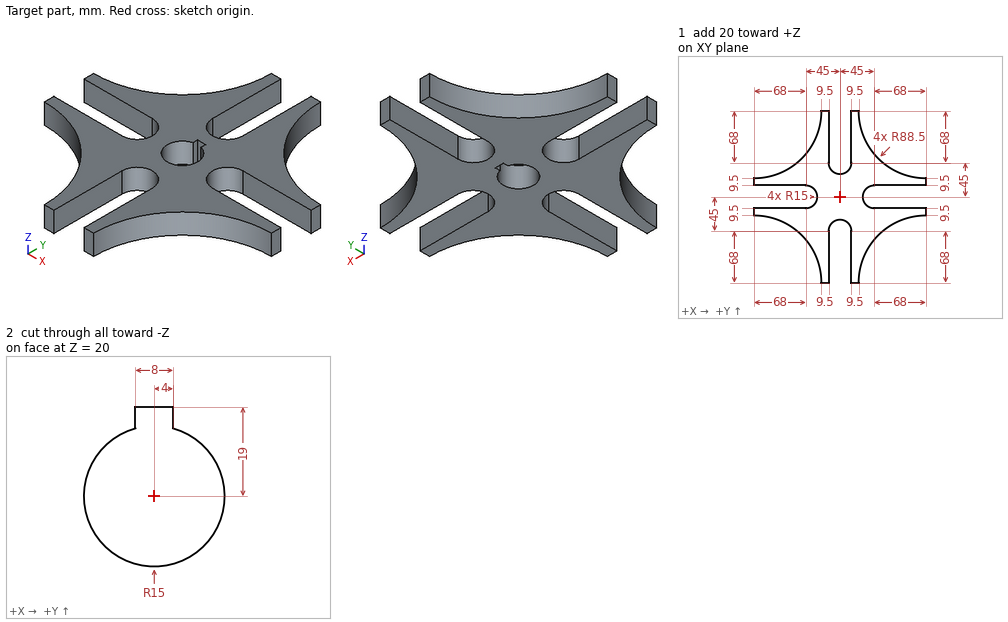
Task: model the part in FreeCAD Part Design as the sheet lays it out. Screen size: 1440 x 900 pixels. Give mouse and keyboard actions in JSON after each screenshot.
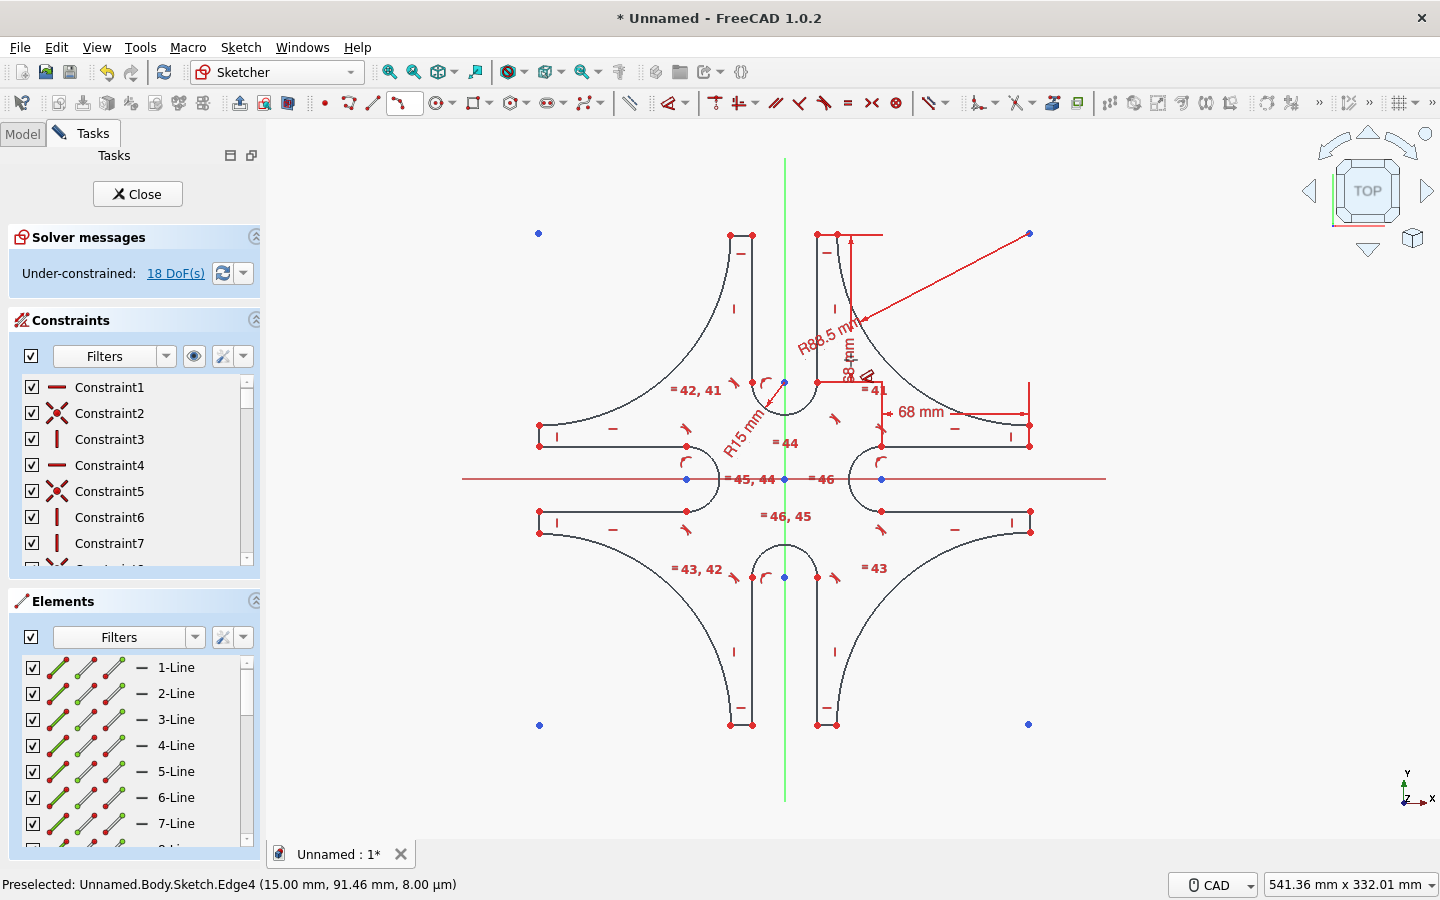
{"action": "left_click", "coordinate": [752, 338]}
{"action": "left_click", "coordinate": [718, 343]}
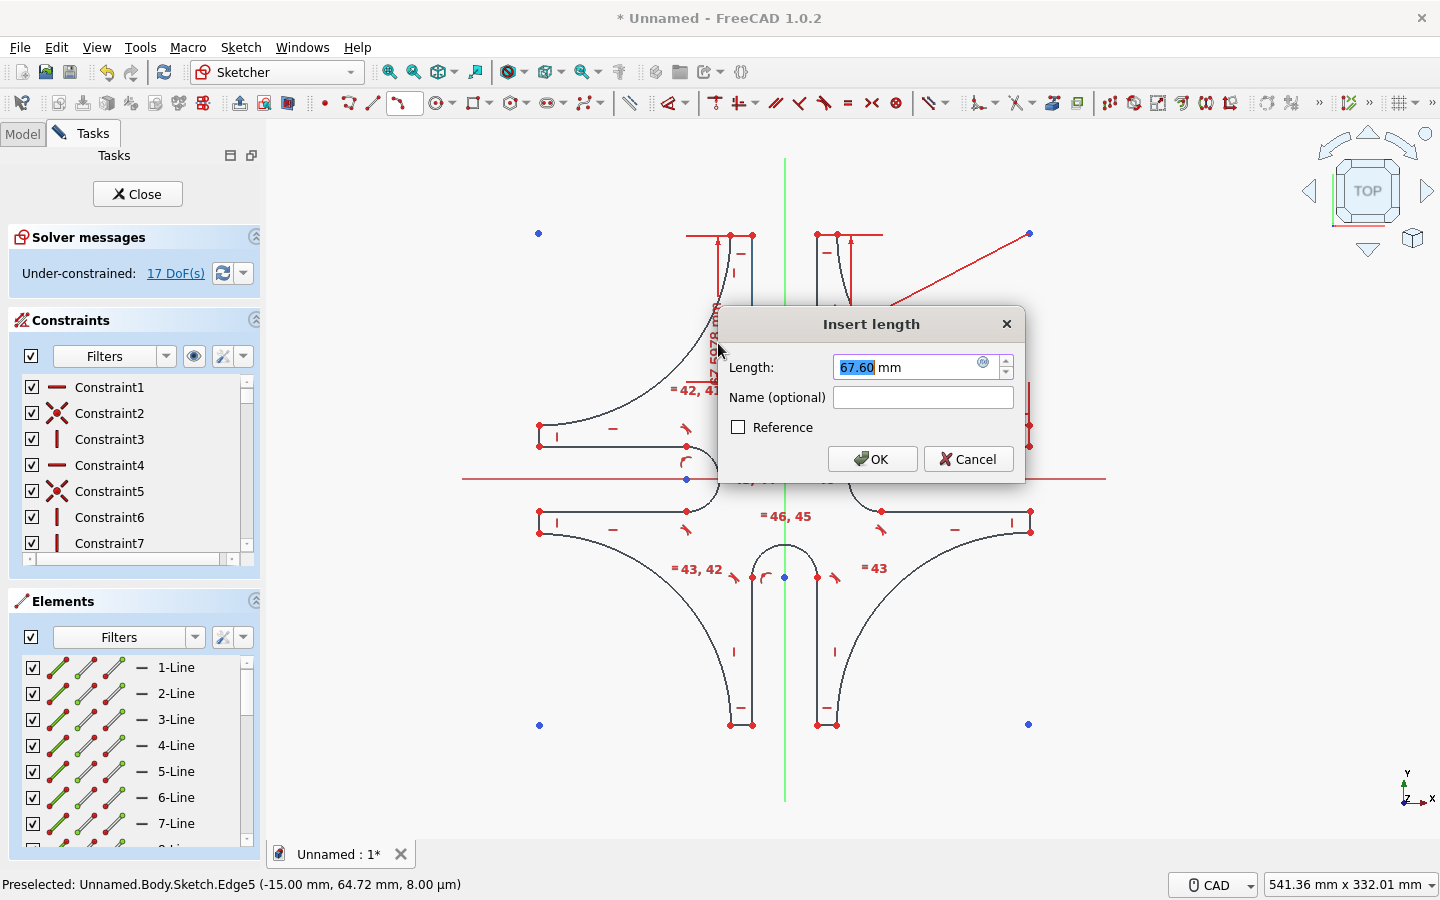
{"action": "type", "text": "68"}
{"action": "key", "text": "Return"}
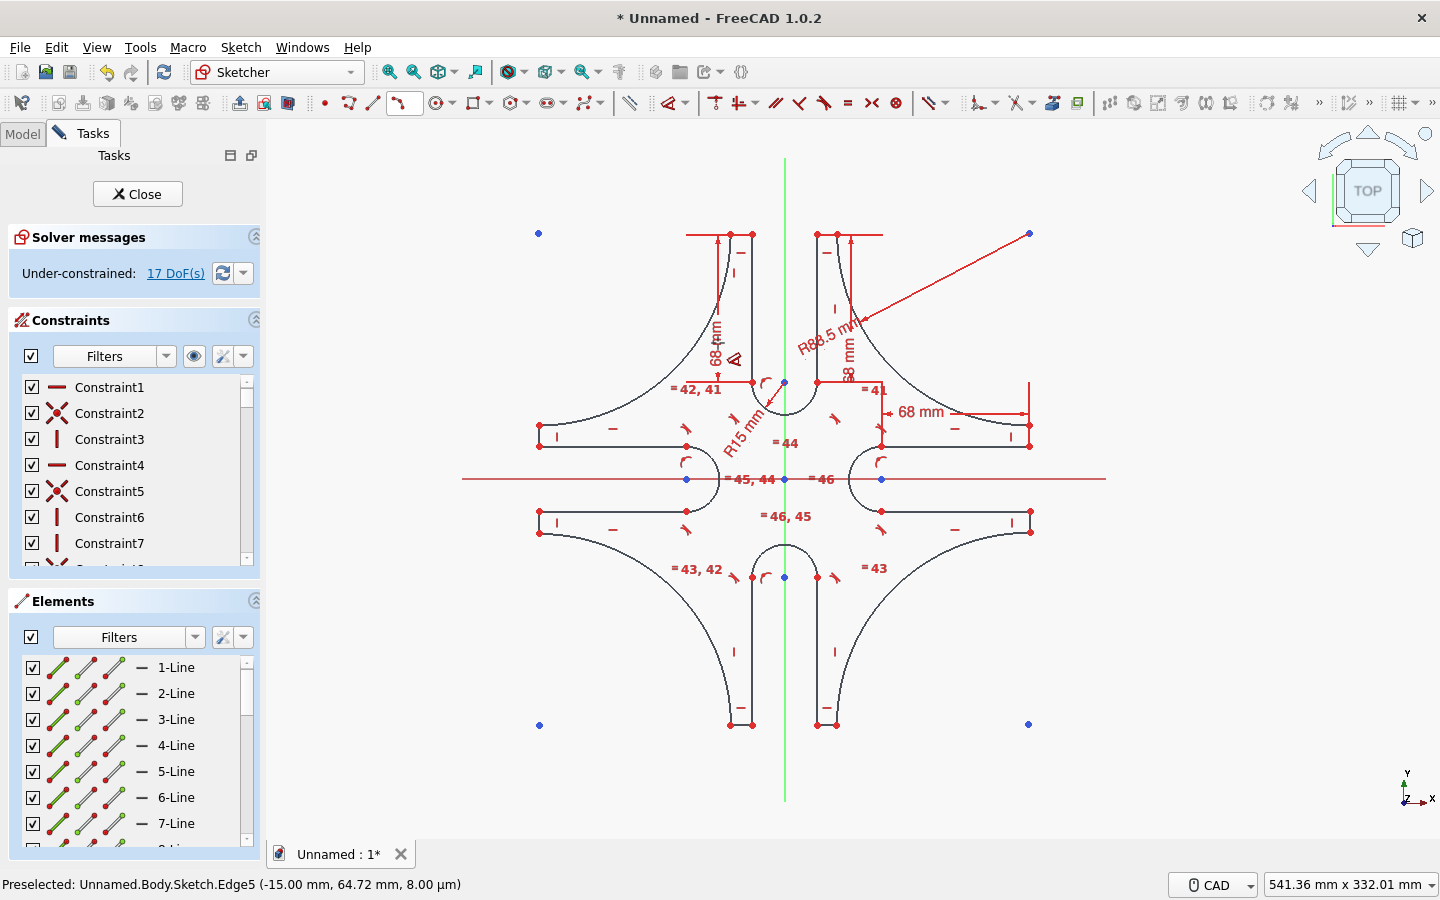
{"action": "left_click", "coordinate": [584, 447]}
{"action": "left_click", "coordinate": [647, 413]}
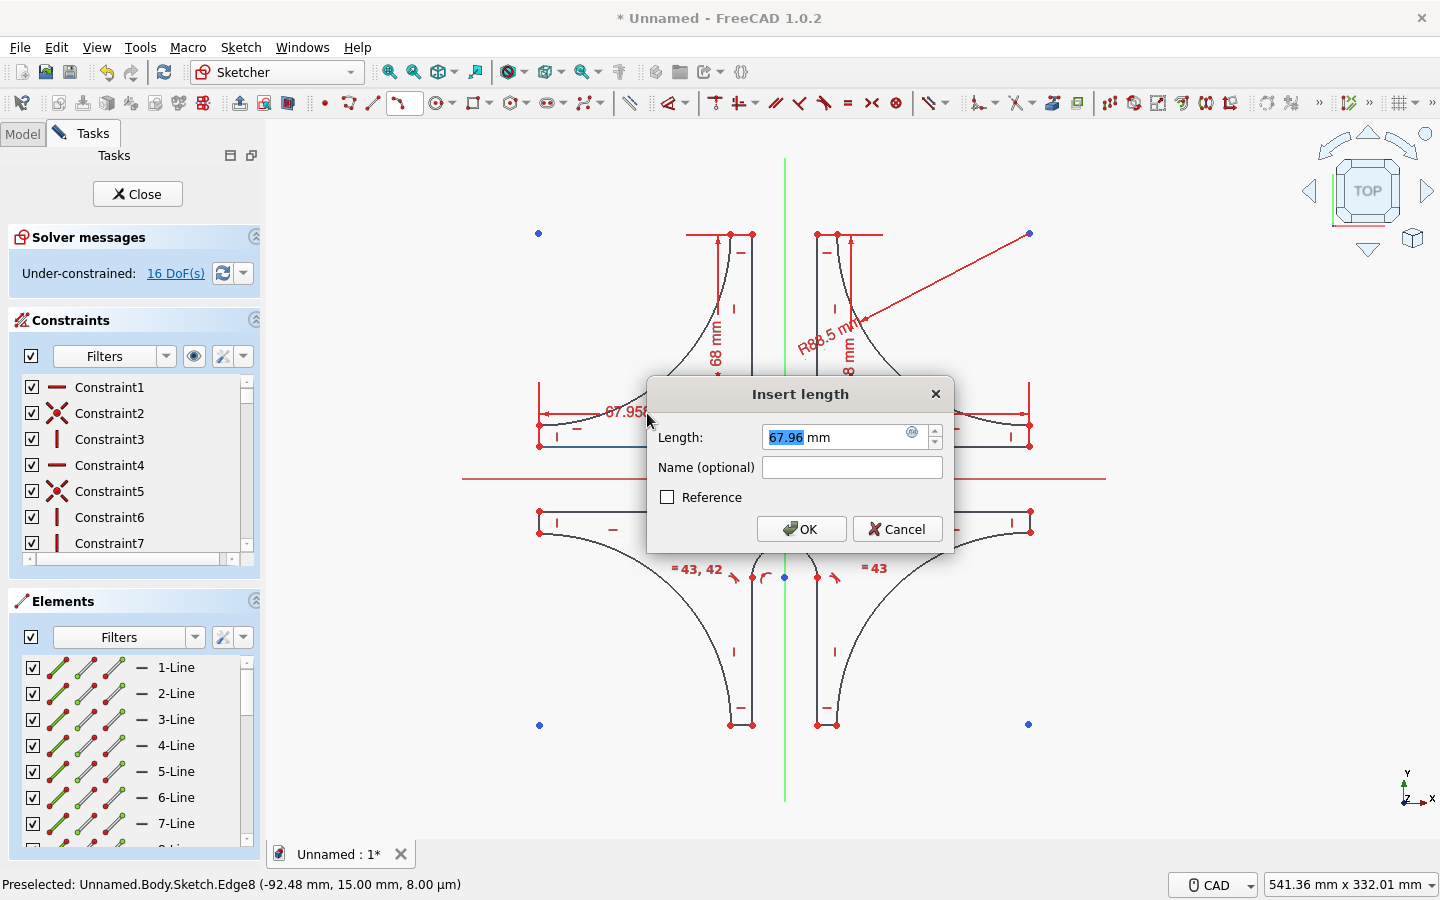
{"action": "type", "text": "68"}
{"action": "key", "text": "Return"}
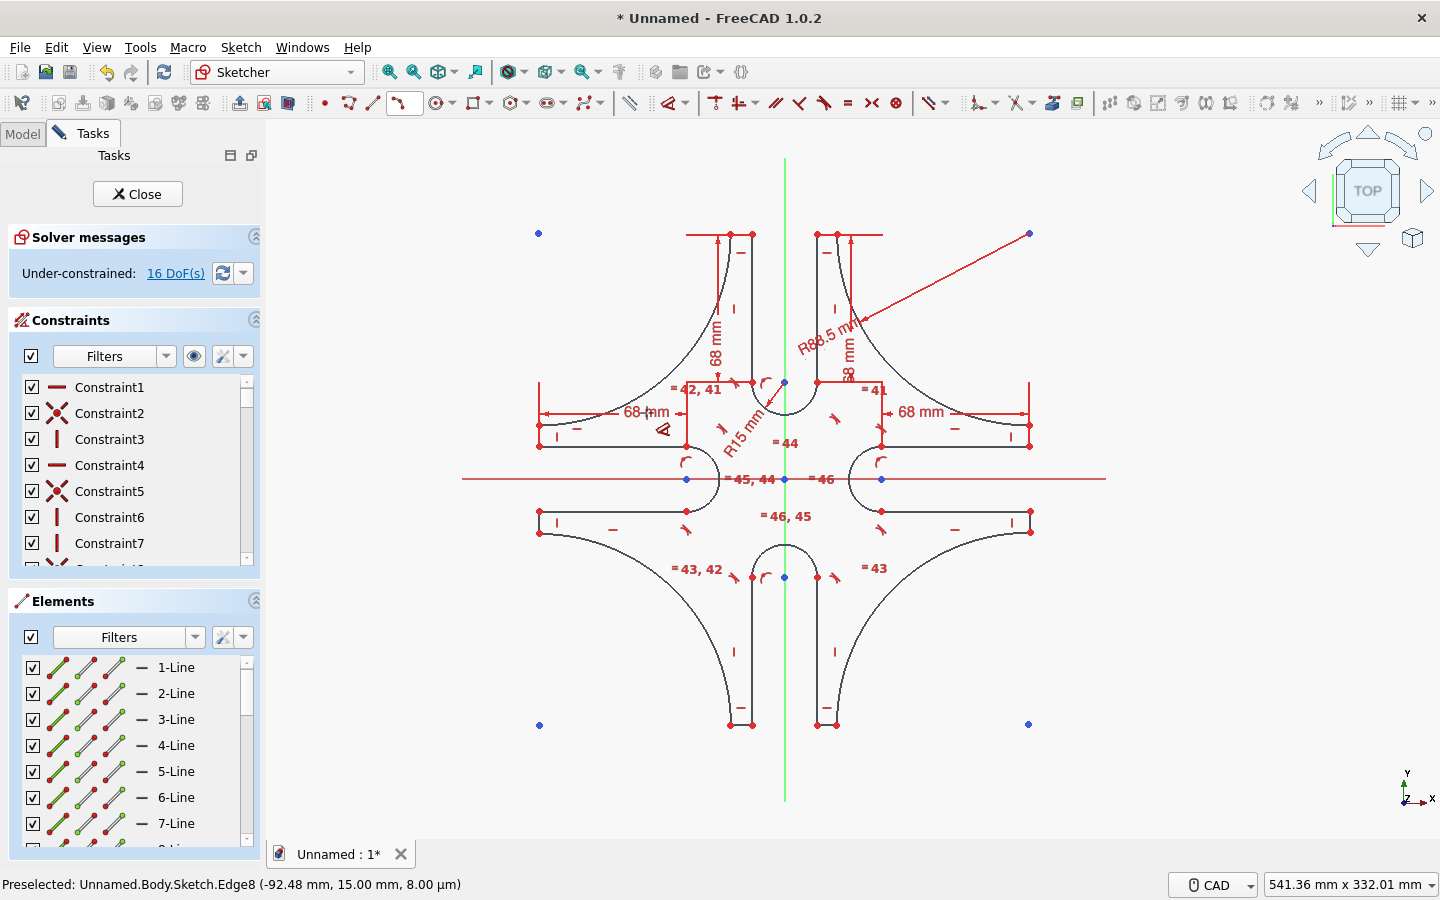
{"action": "left_click", "coordinate": [643, 512]}
{"action": "left_click", "coordinate": [647, 546]}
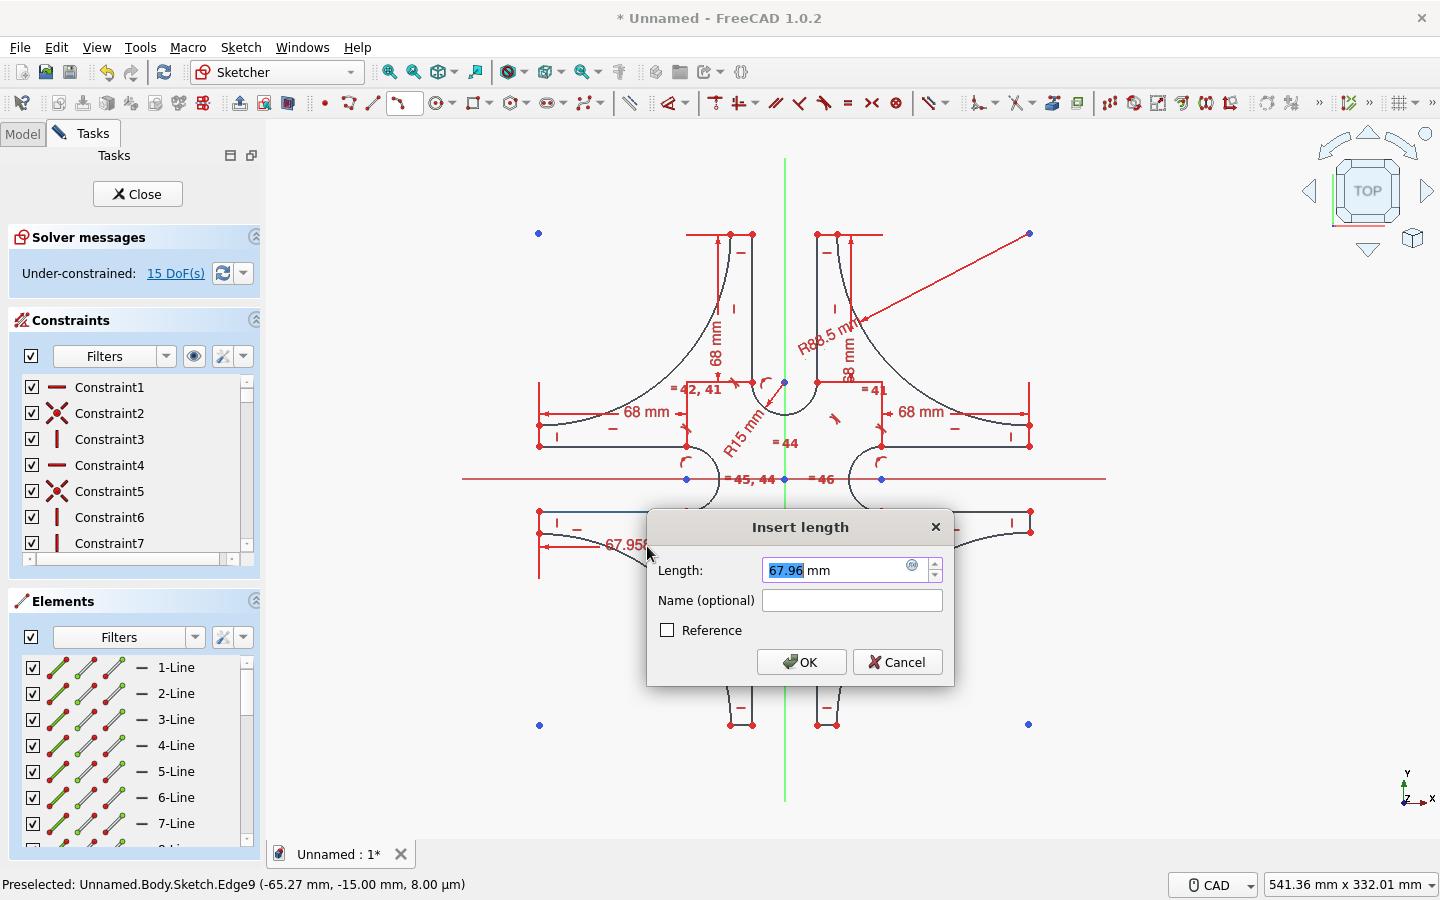
{"action": "type", "text": "68"}
{"action": "key", "text": "Return"}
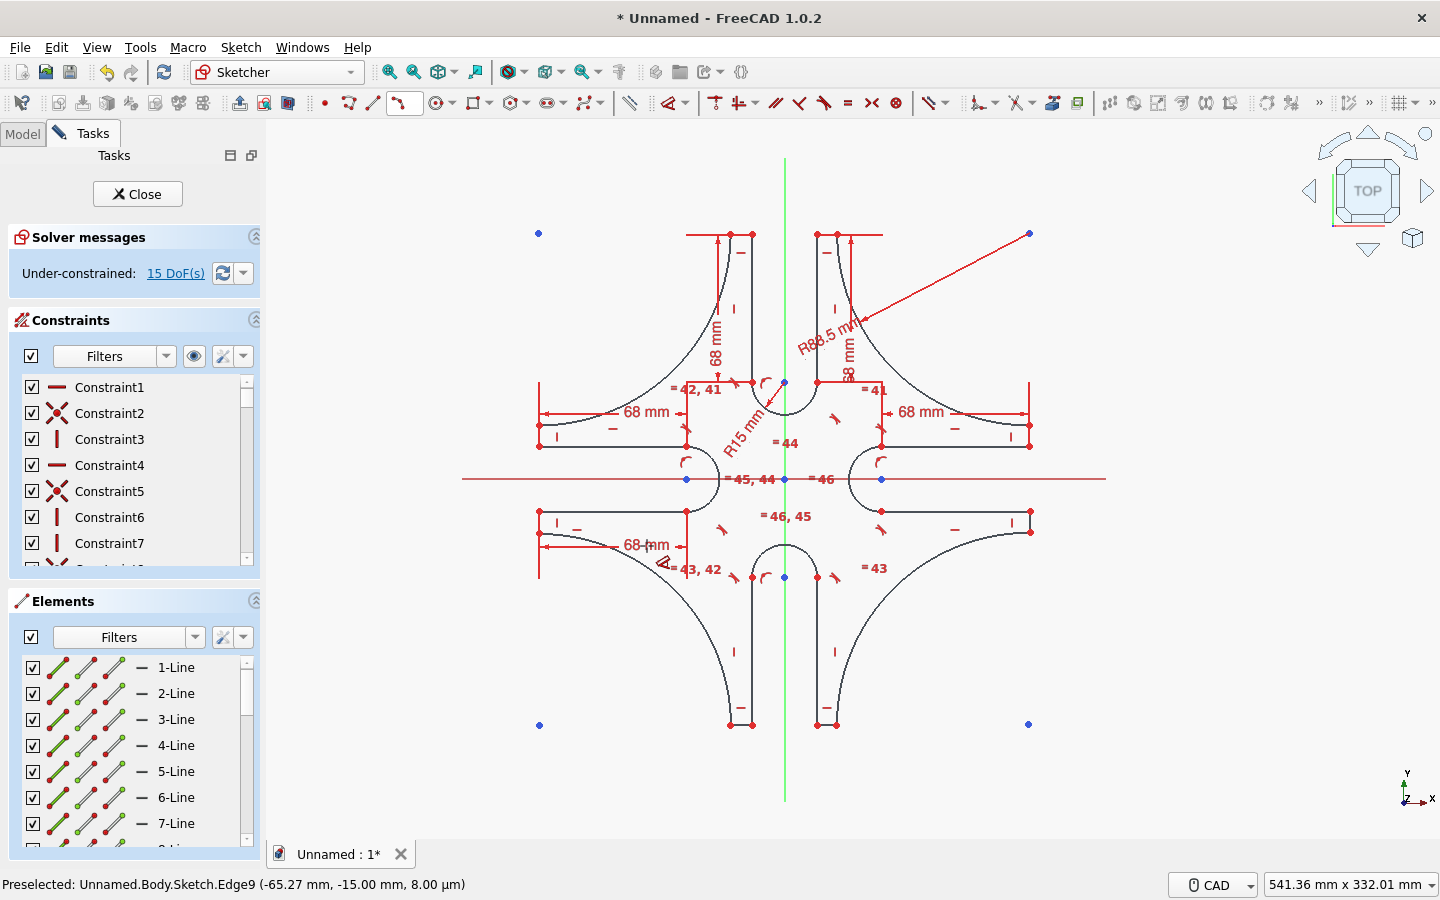
{"action": "left_click", "coordinate": [752, 681]}
{"action": "left_click", "coordinate": [718, 617]}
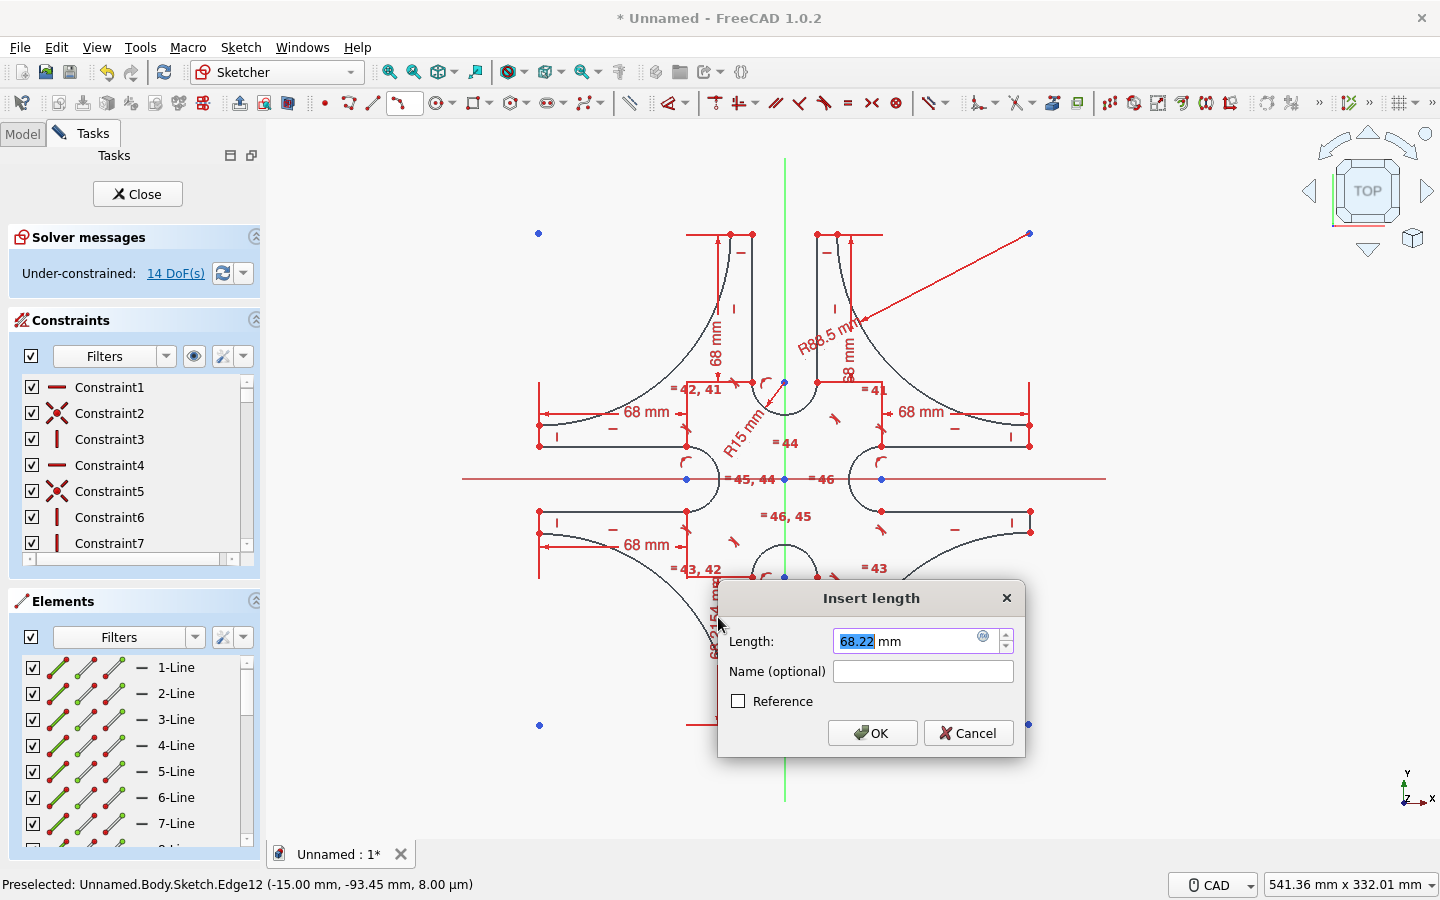
{"action": "type", "text": "68"}
{"action": "key", "text": "Return"}